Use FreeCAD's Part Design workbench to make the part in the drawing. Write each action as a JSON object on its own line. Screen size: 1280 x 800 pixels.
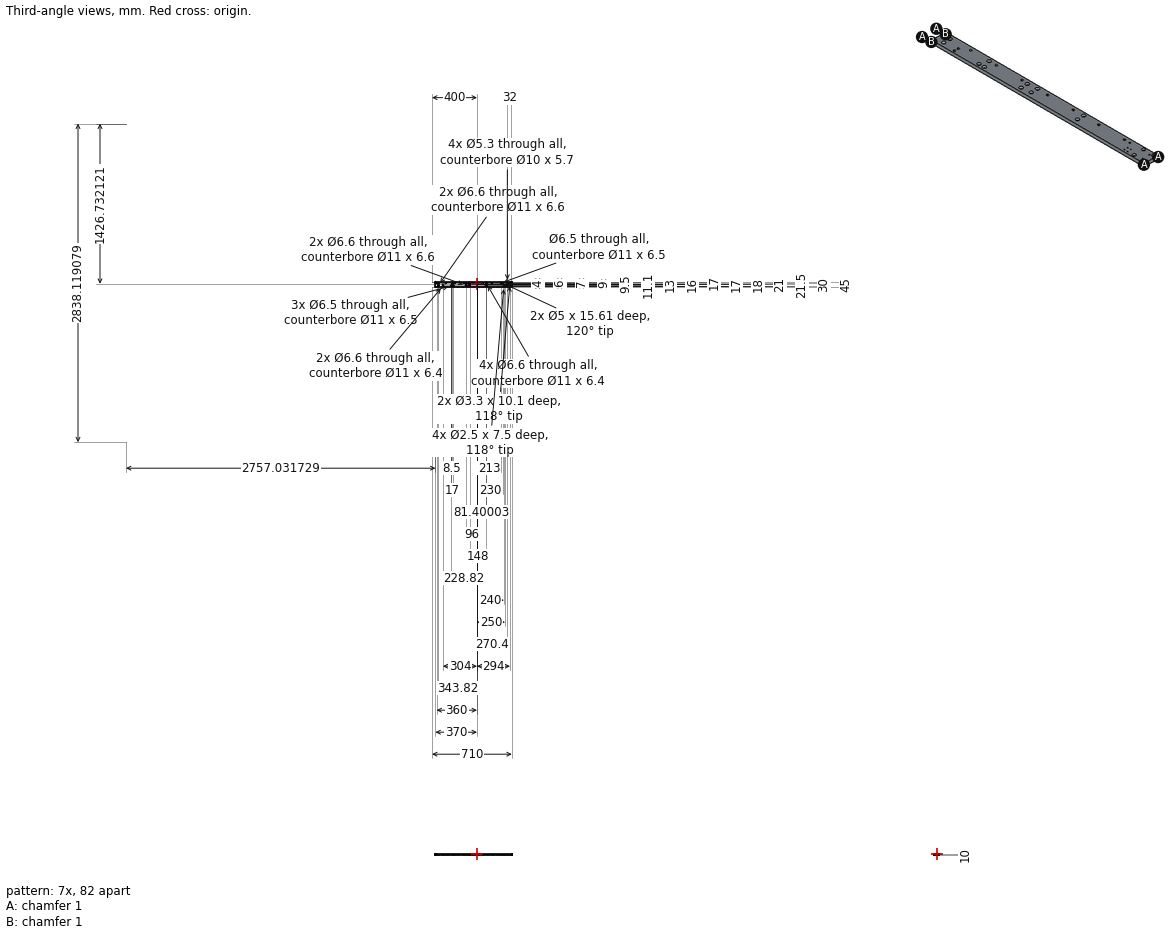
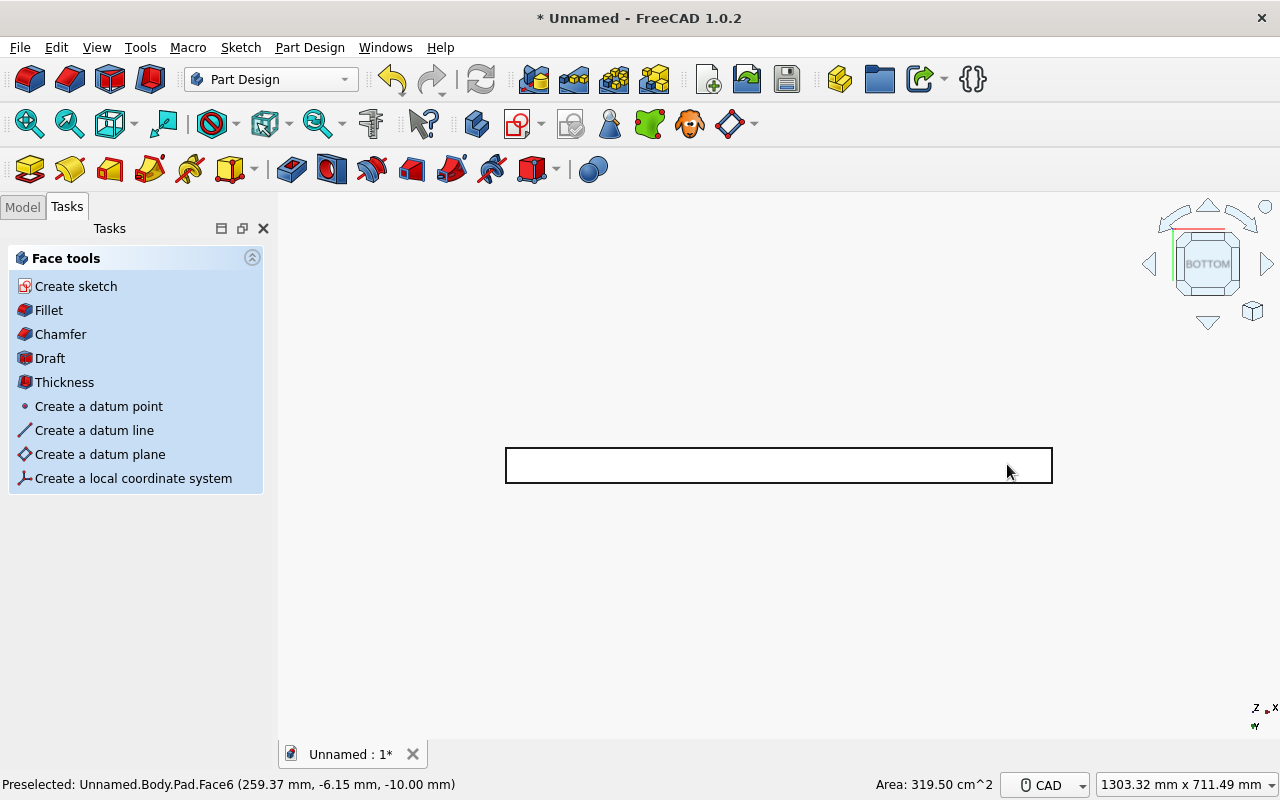
{"action": "left_click", "coordinate": [518, 124]}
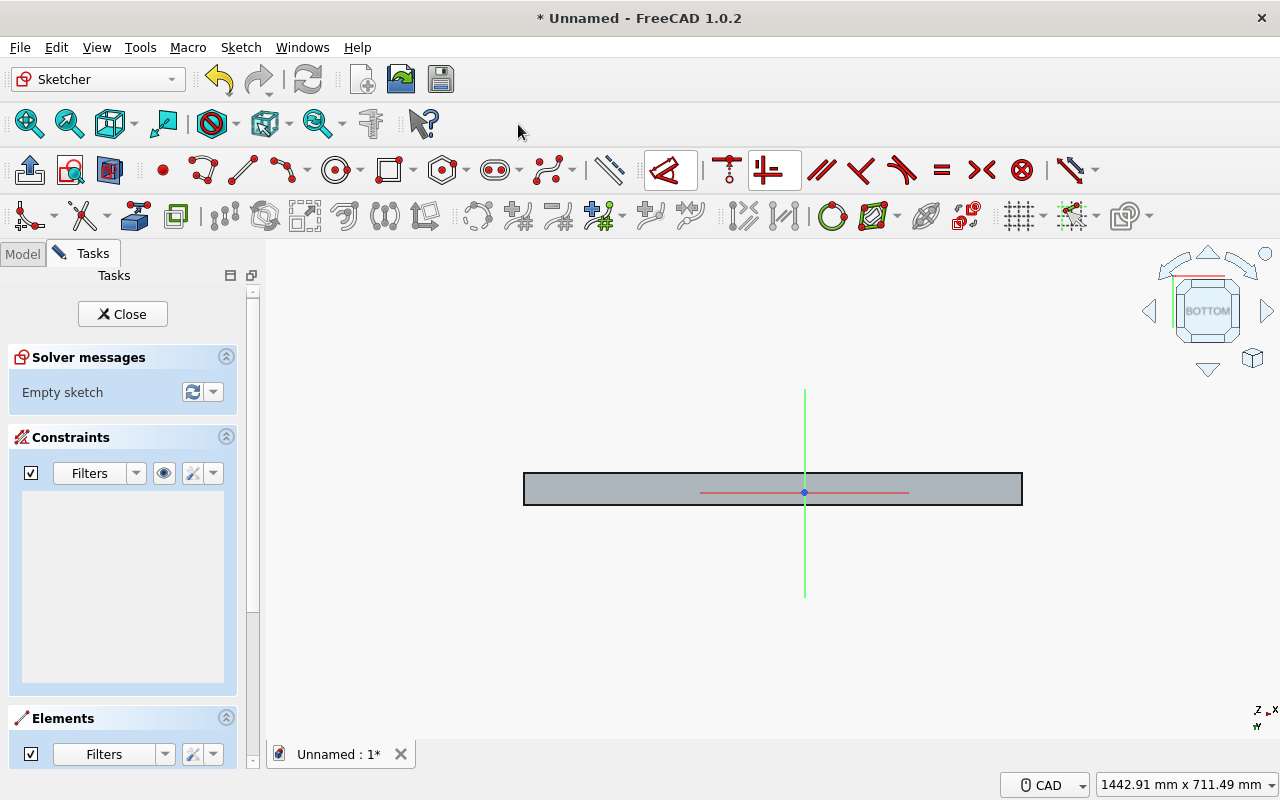
{"action": "scroll", "coordinate": [967, 498], "scroll_direction": "up", "scroll_amount": 15}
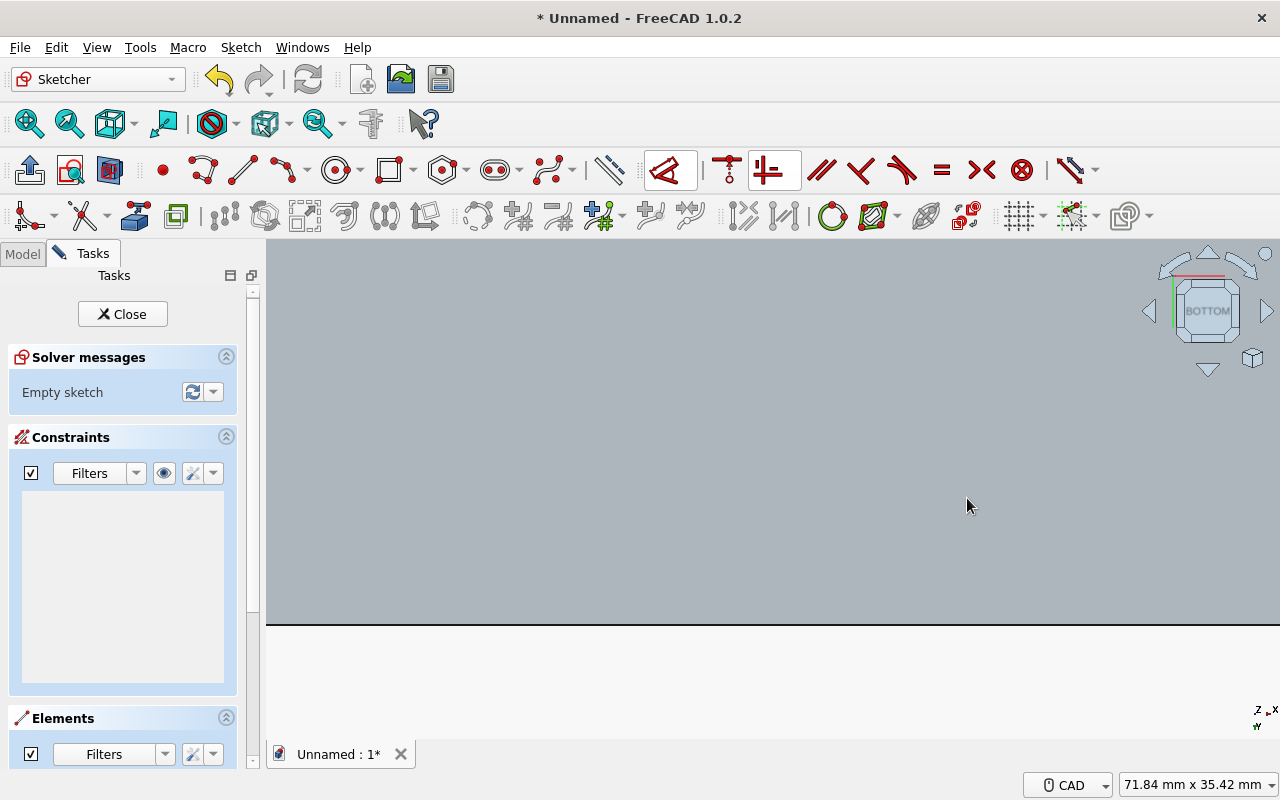
{"action": "scroll", "coordinate": [696, 461], "scroll_direction": "up", "scroll_amount": 6}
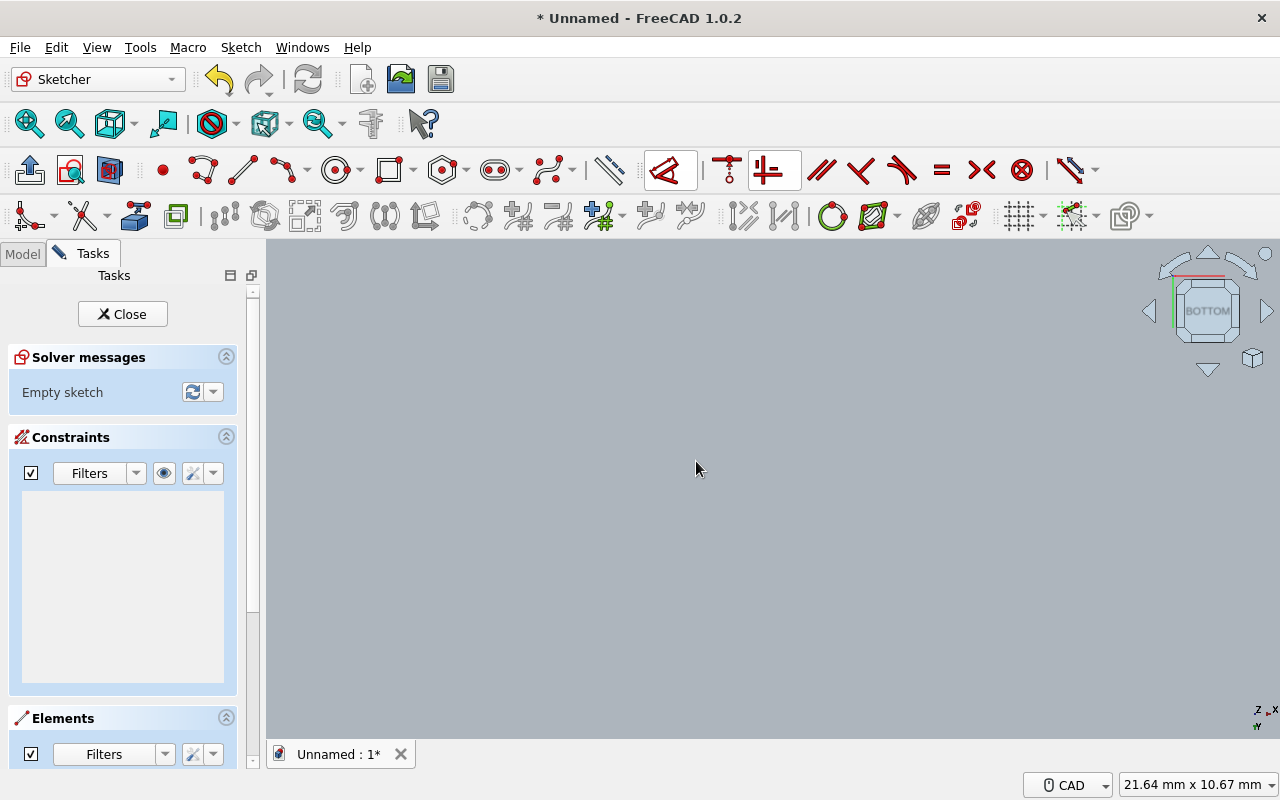
{"action": "left_click", "coordinate": [336, 170]}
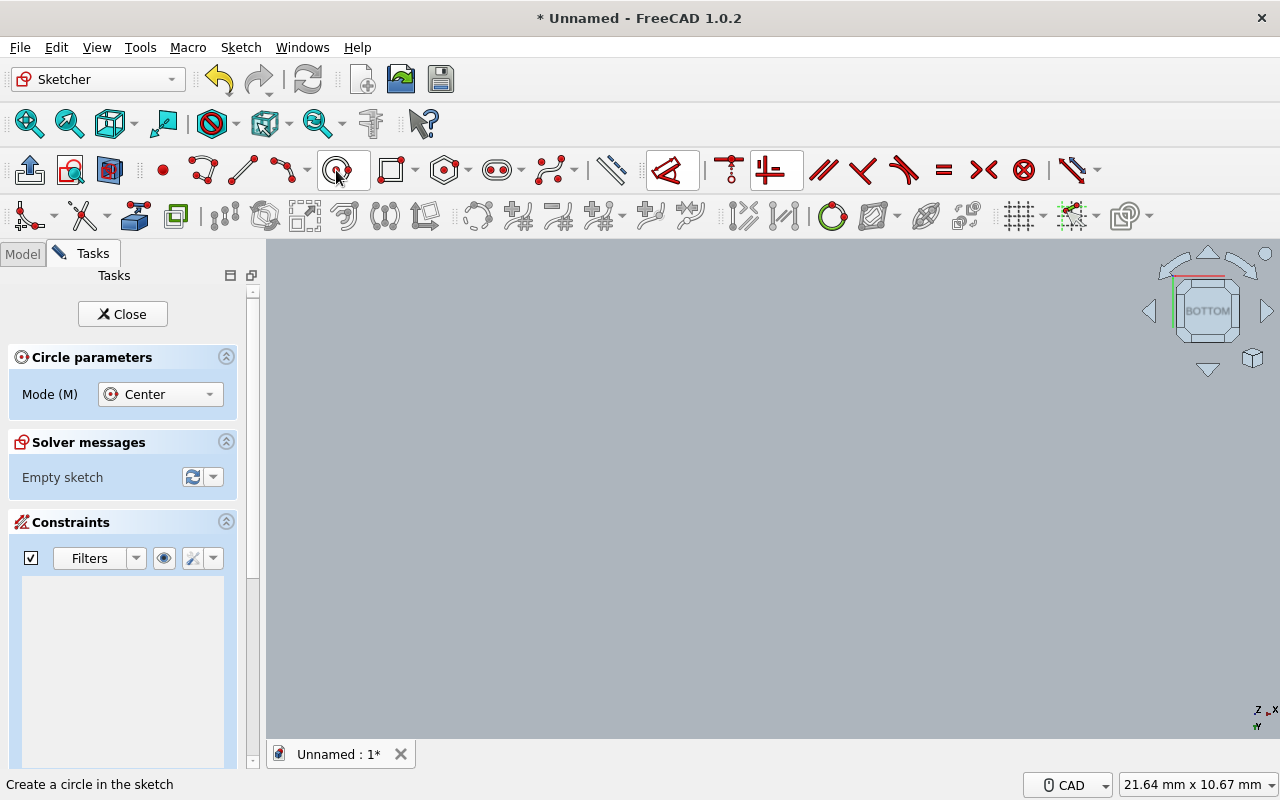
{"action": "left_click", "coordinate": [705, 489]}
{"action": "left_click", "coordinate": [812, 381]}
{"action": "key", "text": "Escape"}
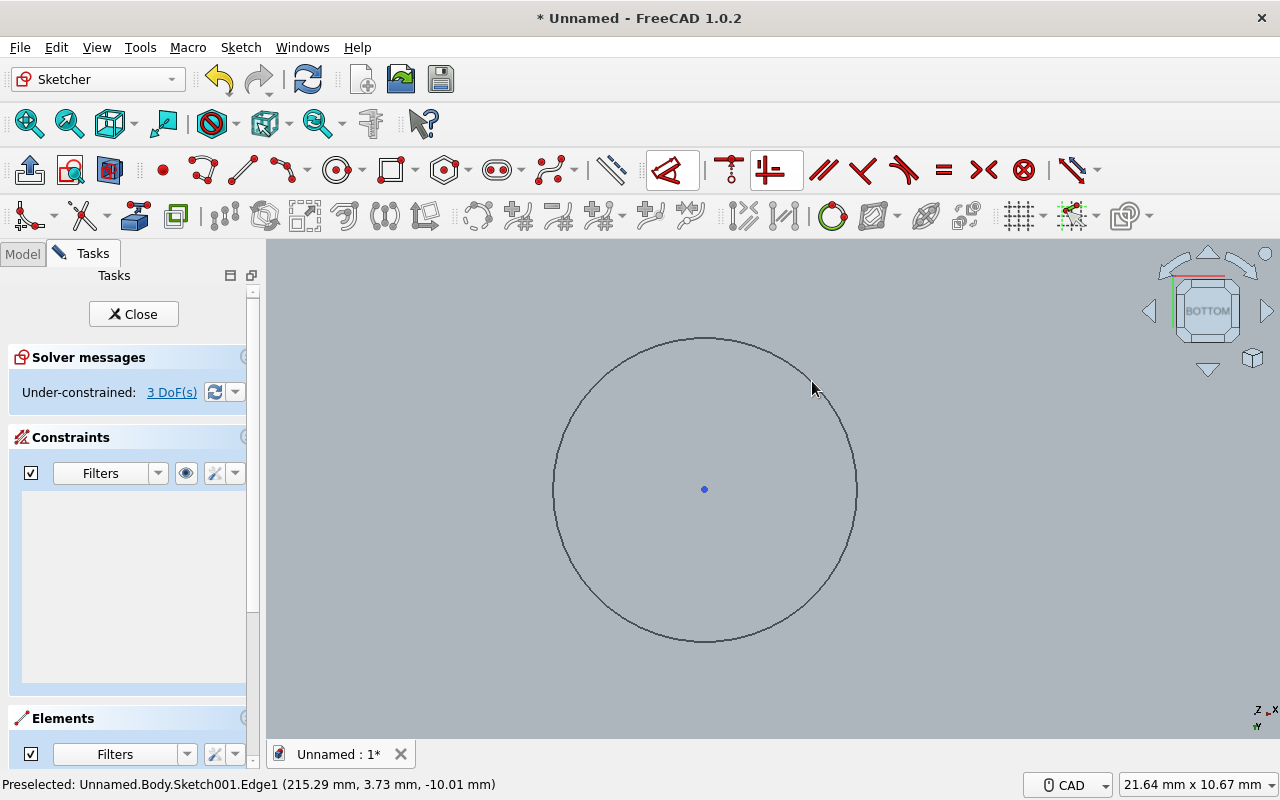
{"action": "left_click", "coordinate": [812, 382]}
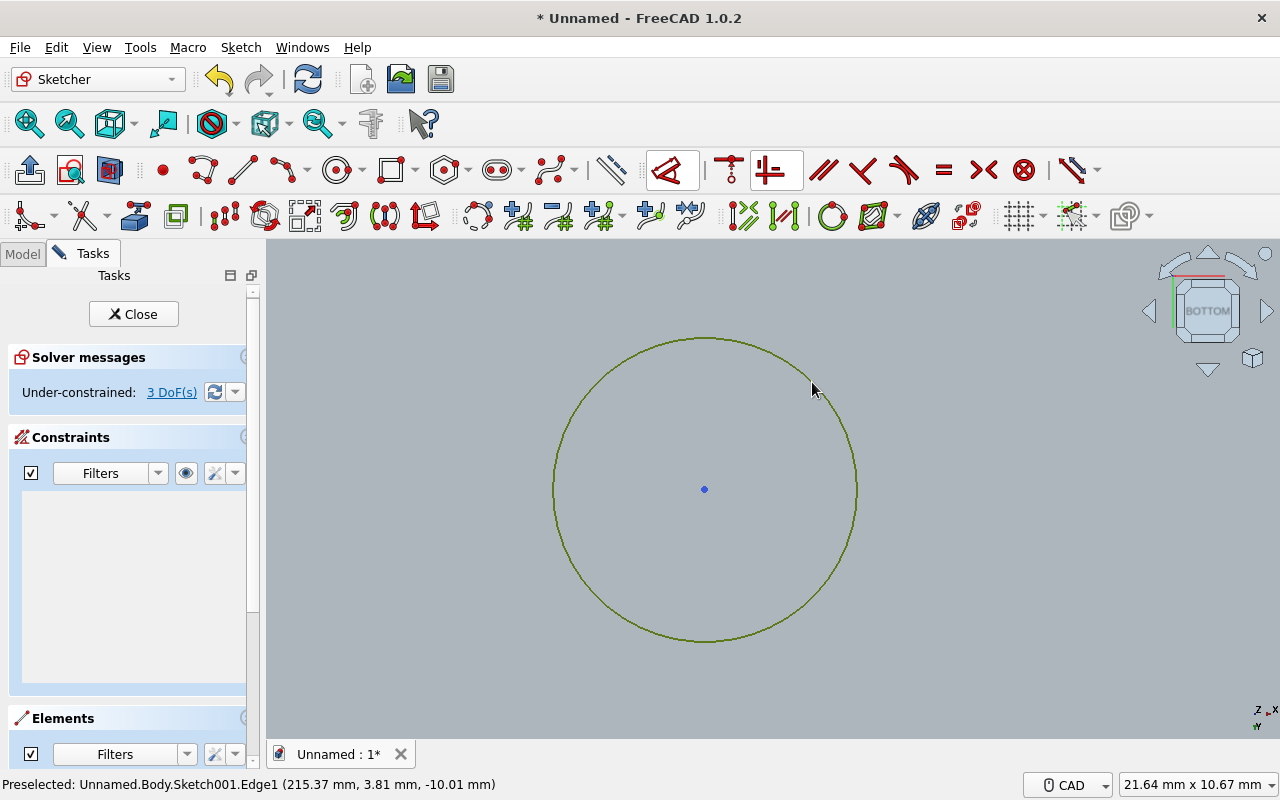
{"action": "left_click", "coordinate": [694, 170]}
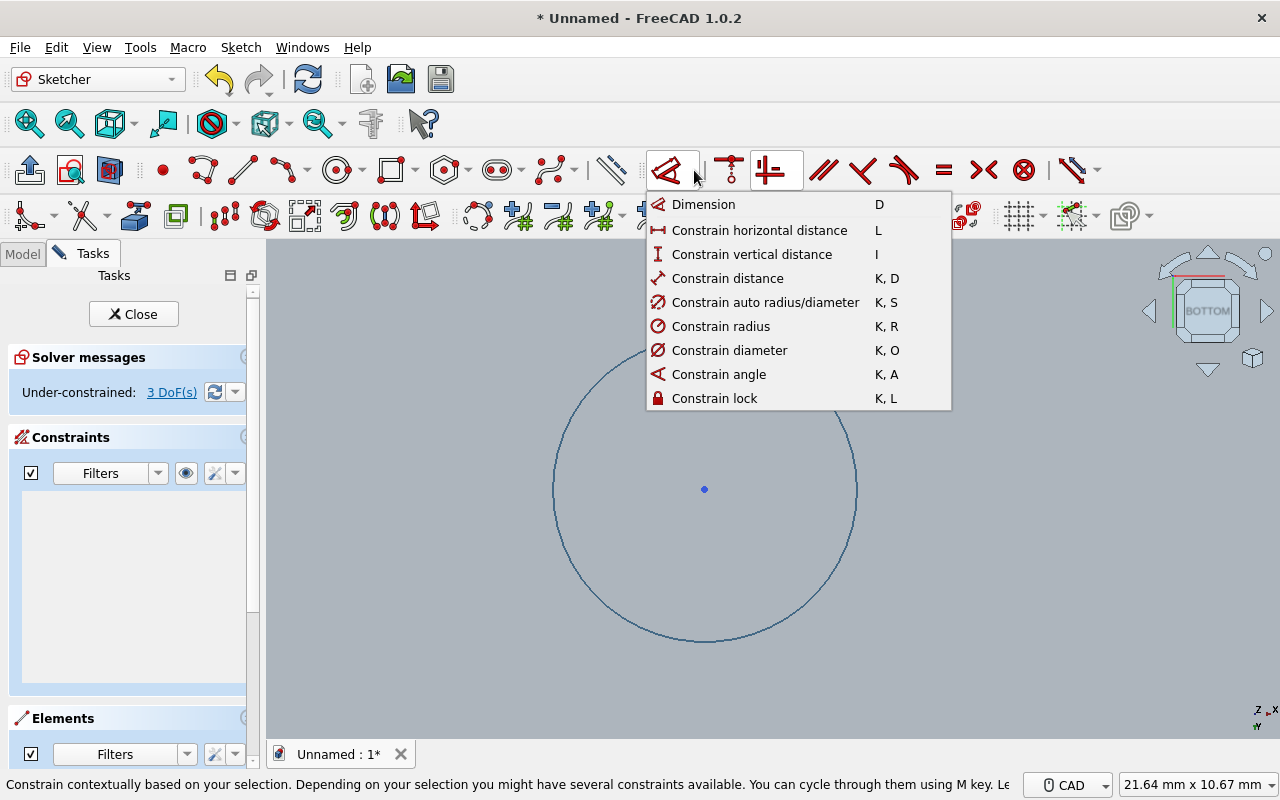
{"action": "left_click", "coordinate": [799, 350]}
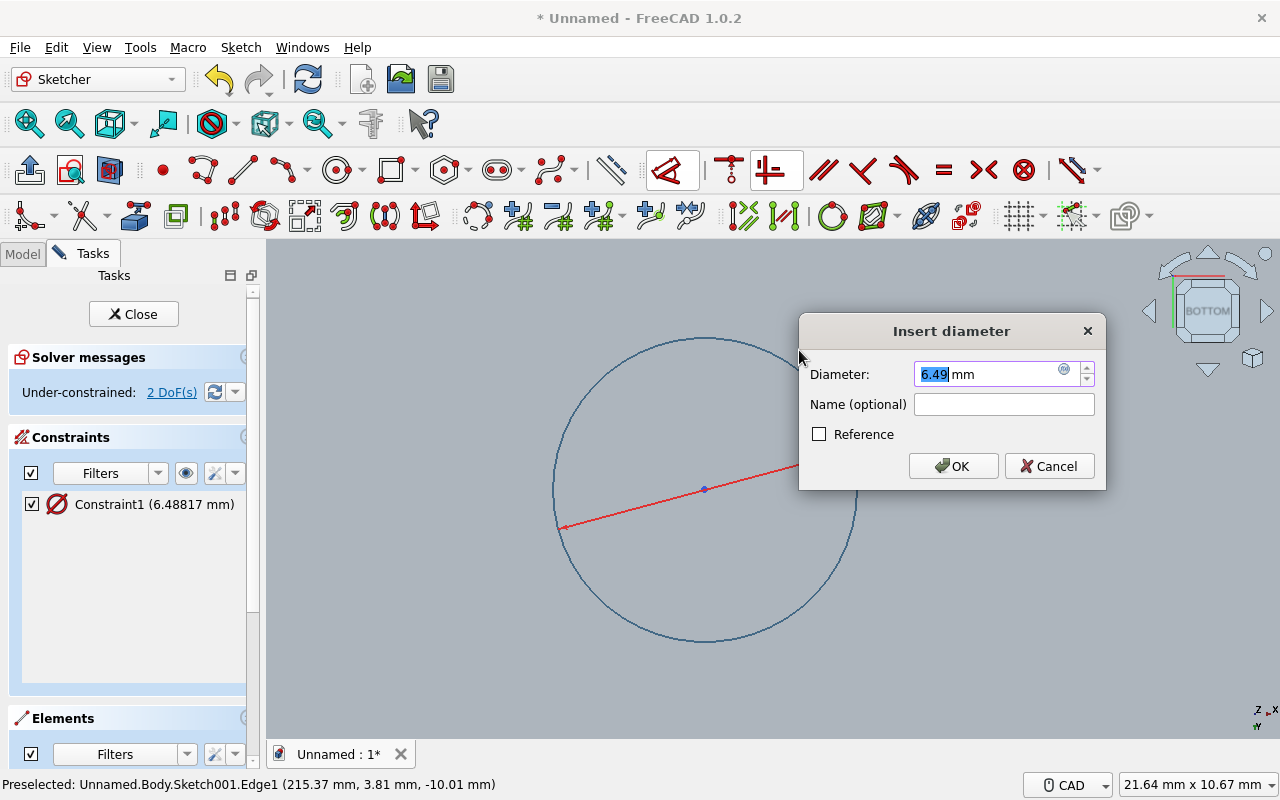
{"action": "type", "text": "6.5"}
{"action": "key", "text": "Return"}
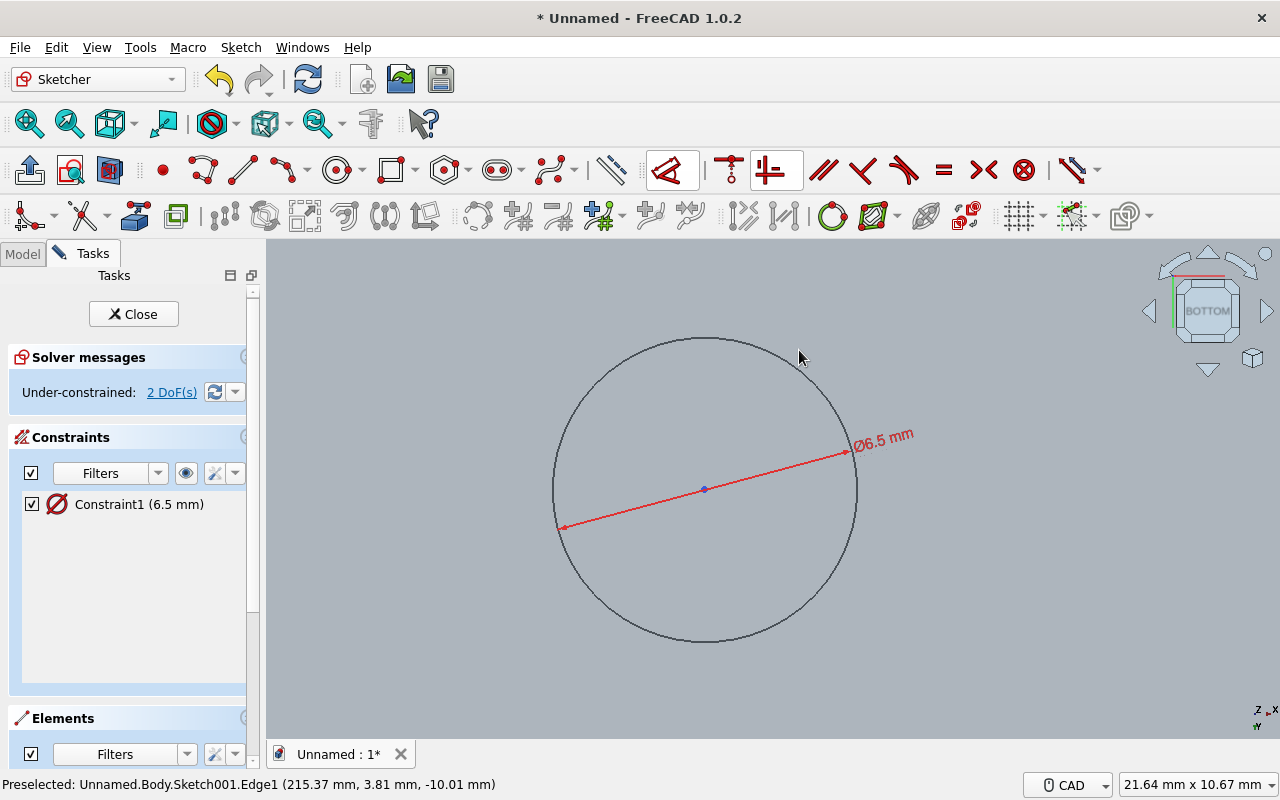
{"action": "left_click", "coordinate": [705, 490]}